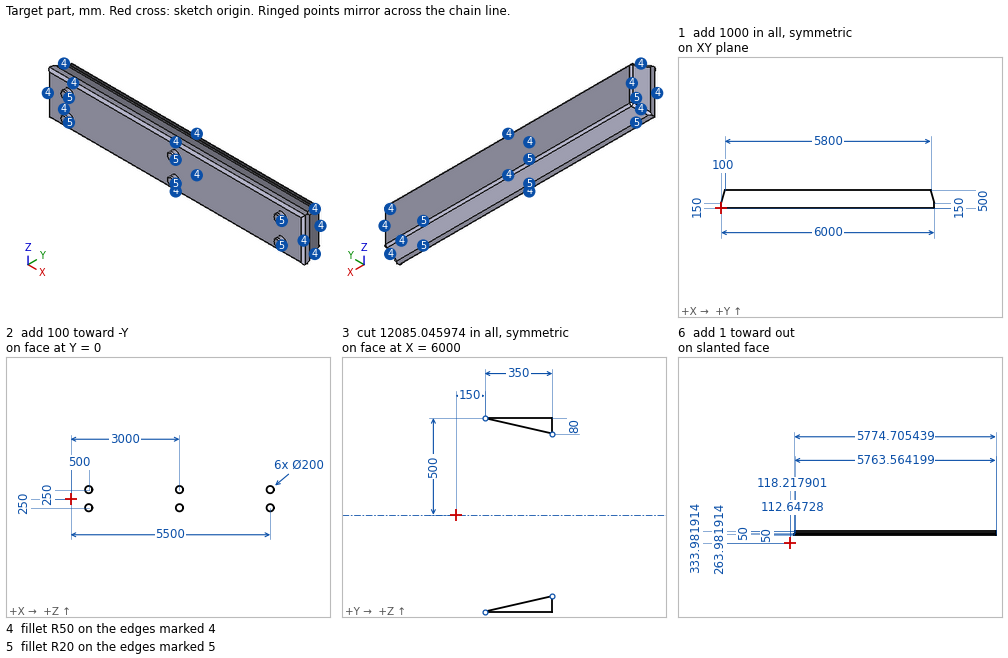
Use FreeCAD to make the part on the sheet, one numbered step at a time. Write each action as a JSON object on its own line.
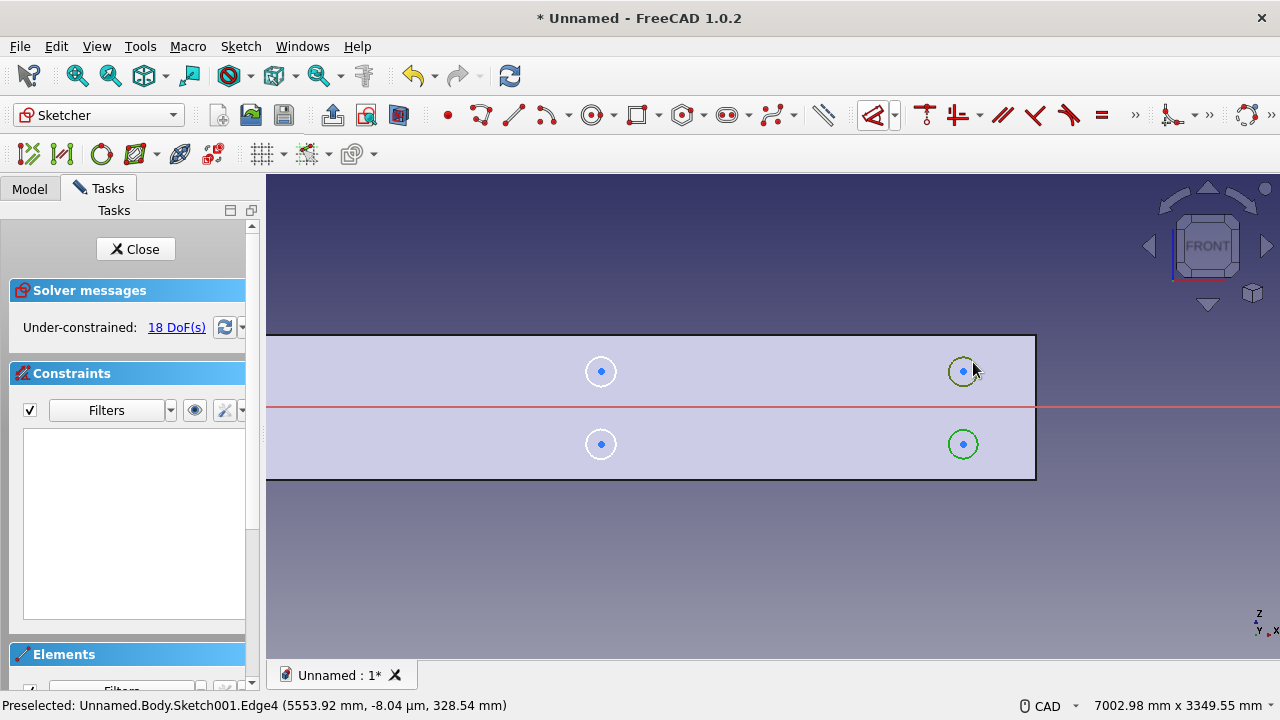
{"action": "left_click", "coordinate": [611, 361]}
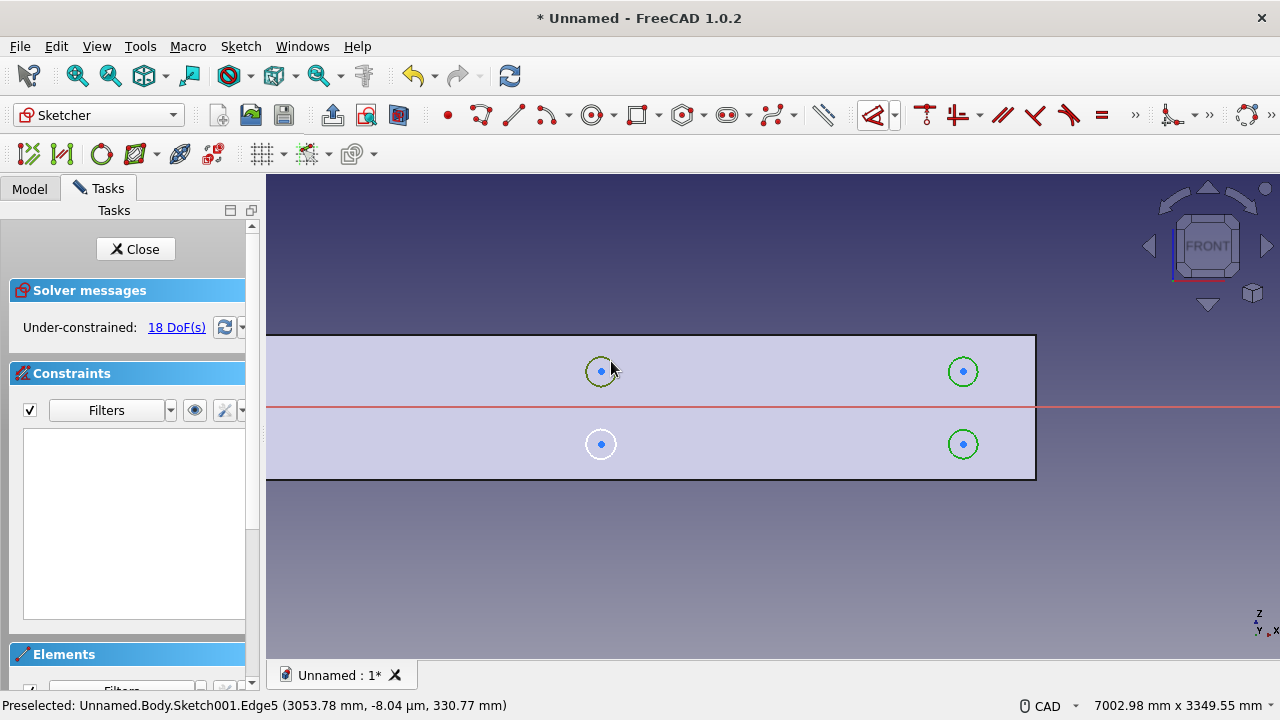
{"action": "left_click", "coordinate": [611, 434]}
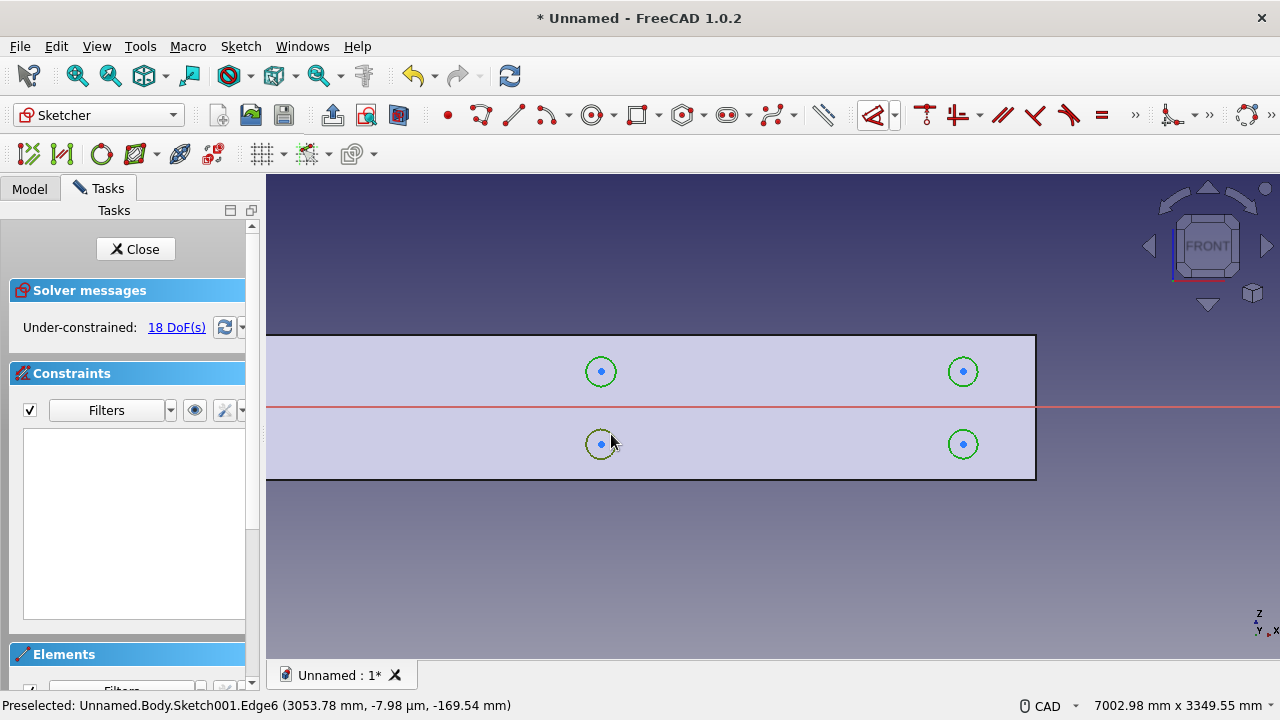
{"action": "left_click", "coordinate": [1102, 116]}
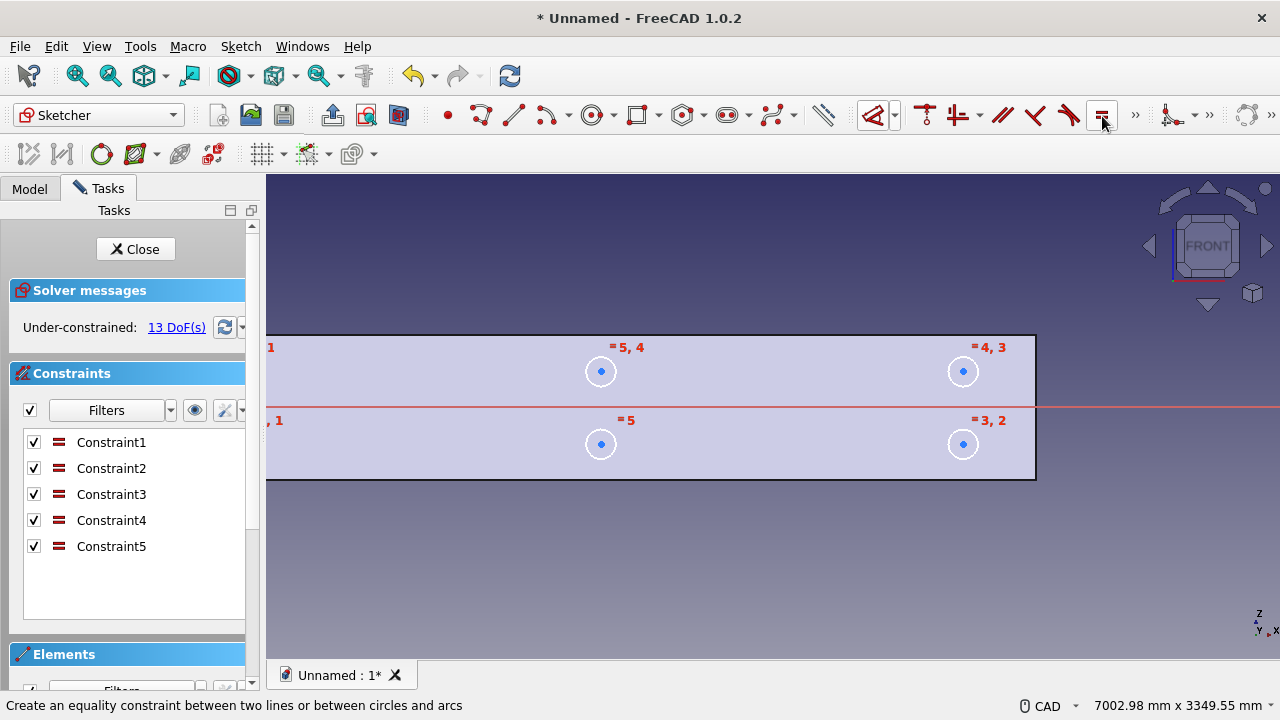
{"action": "scroll", "coordinate": [974, 435], "scroll_direction": "down", "scroll_amount": 2}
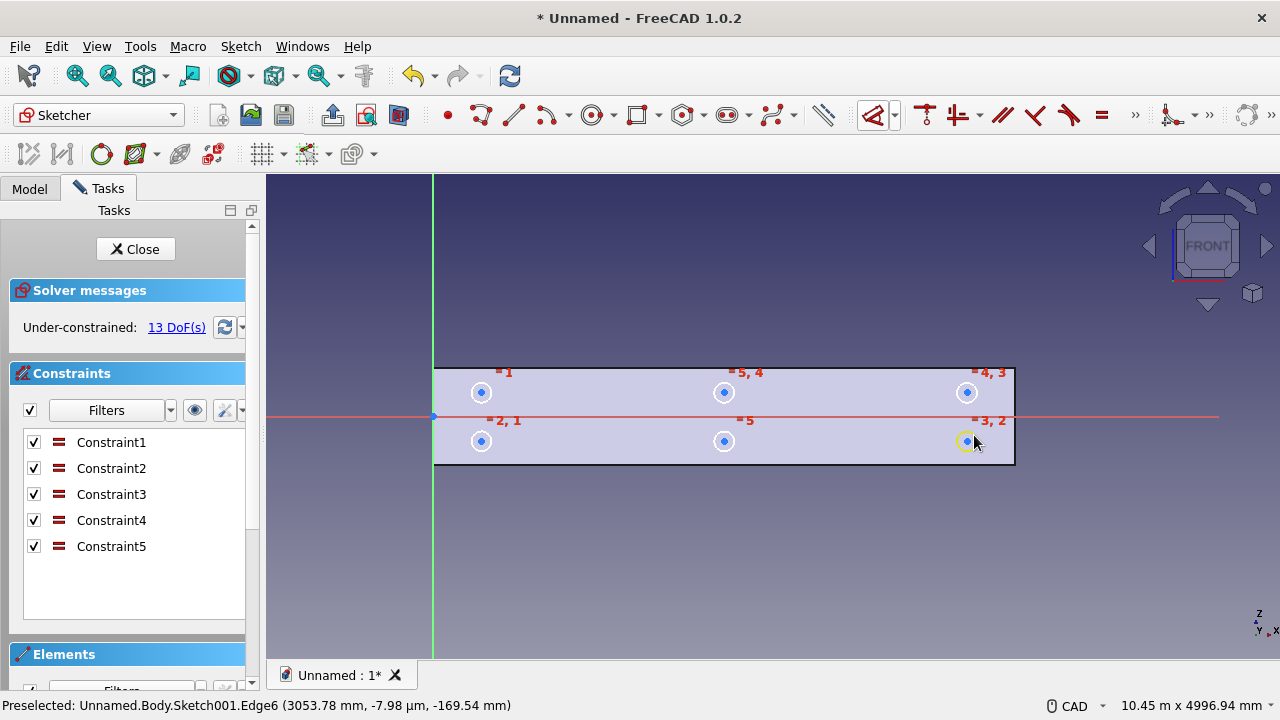
{"action": "left_click", "coordinate": [481, 393]}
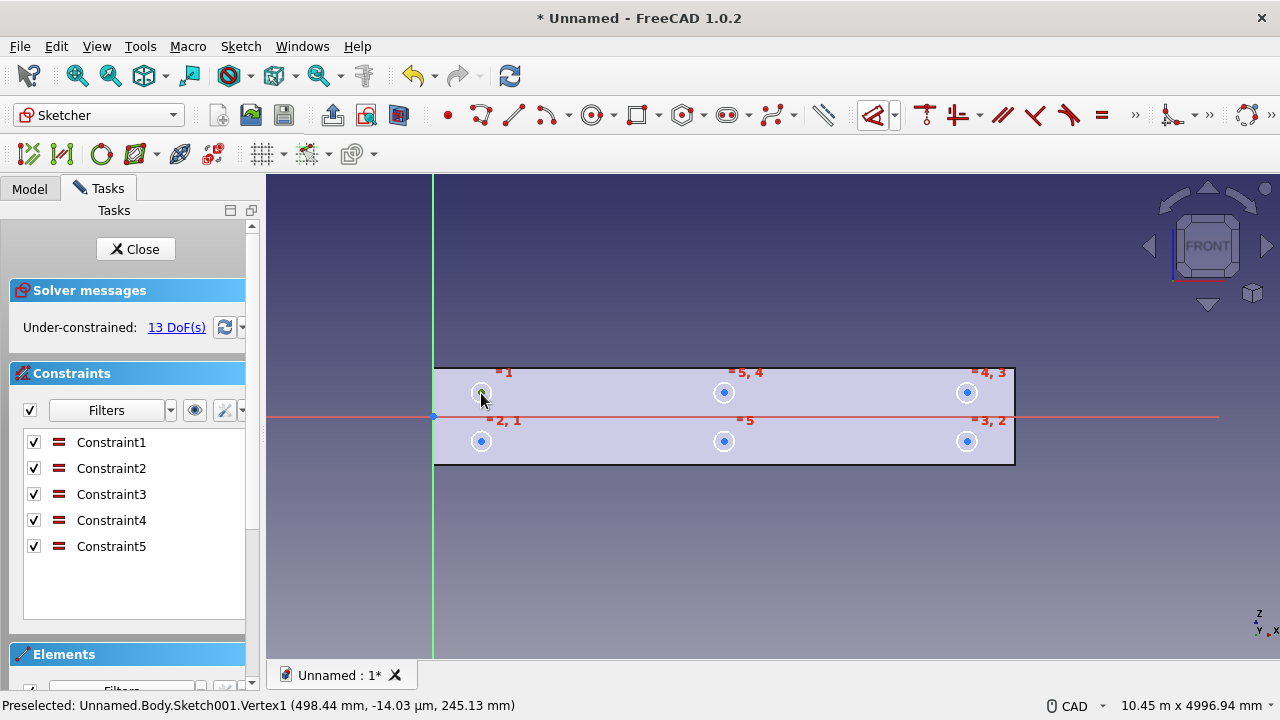
{"action": "left_click", "coordinate": [481, 441]}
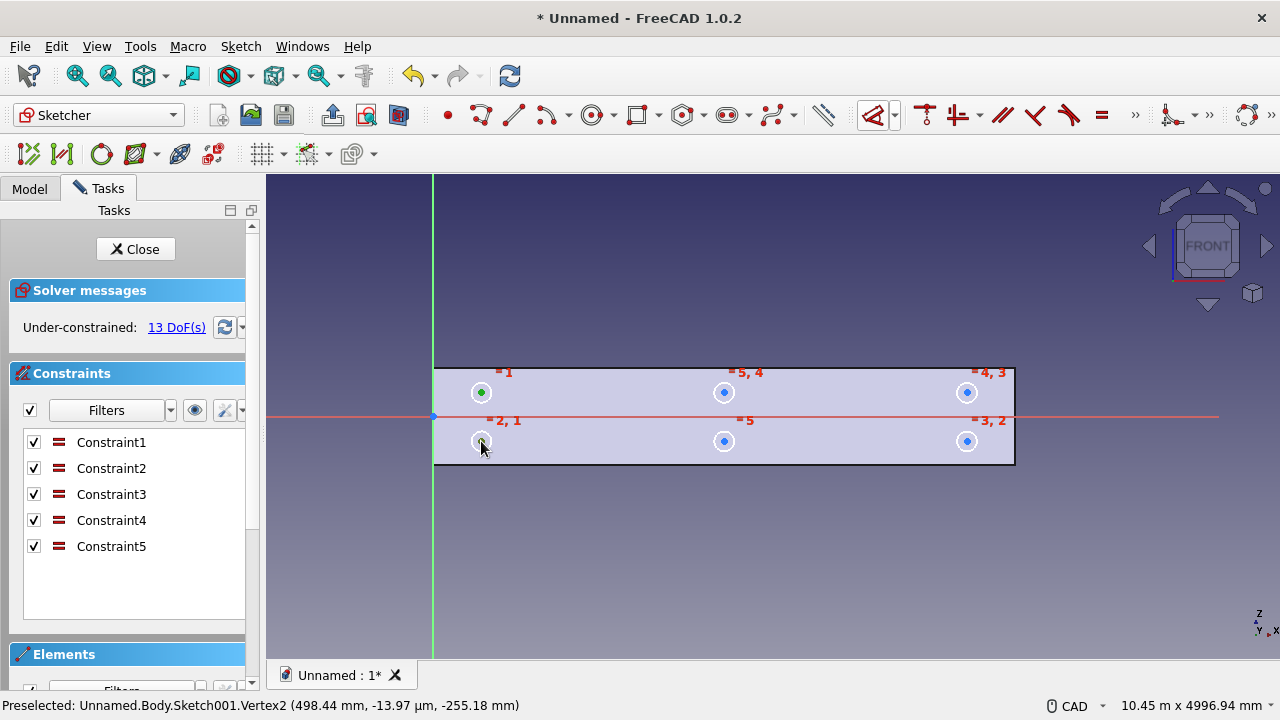
{"action": "left_click", "coordinate": [980, 116]}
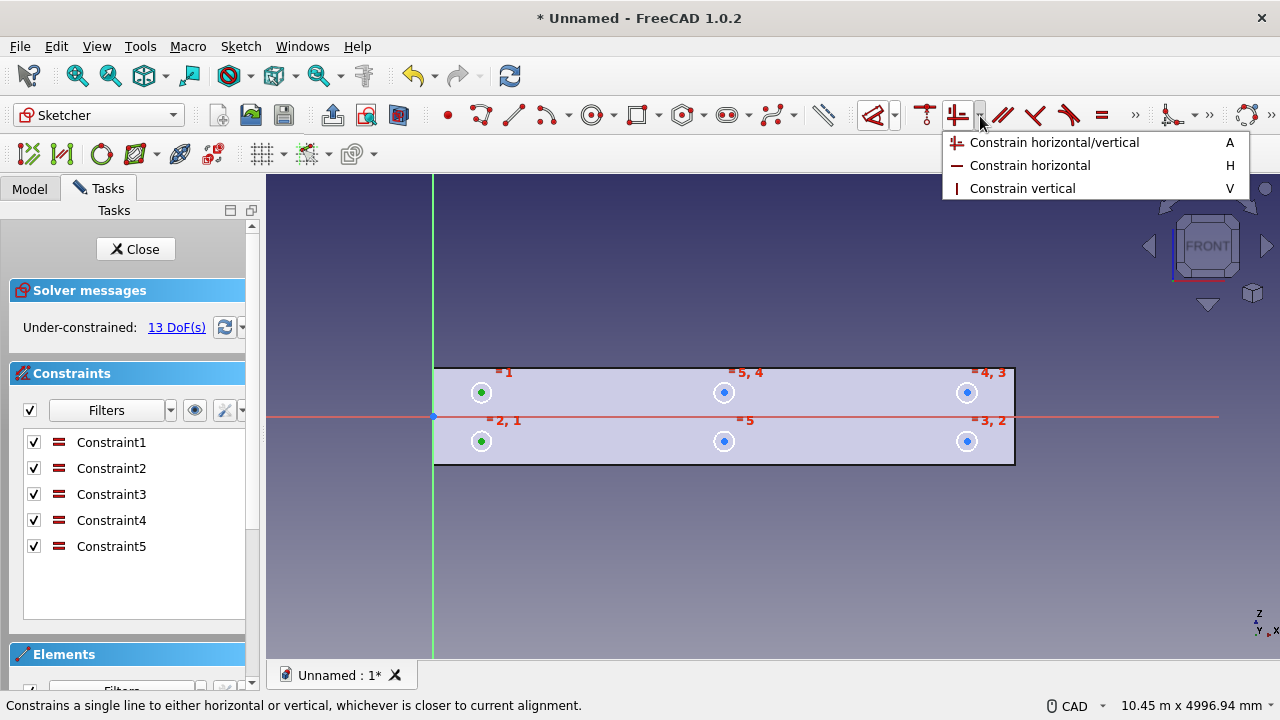
{"action": "left_click", "coordinate": [1096, 188]}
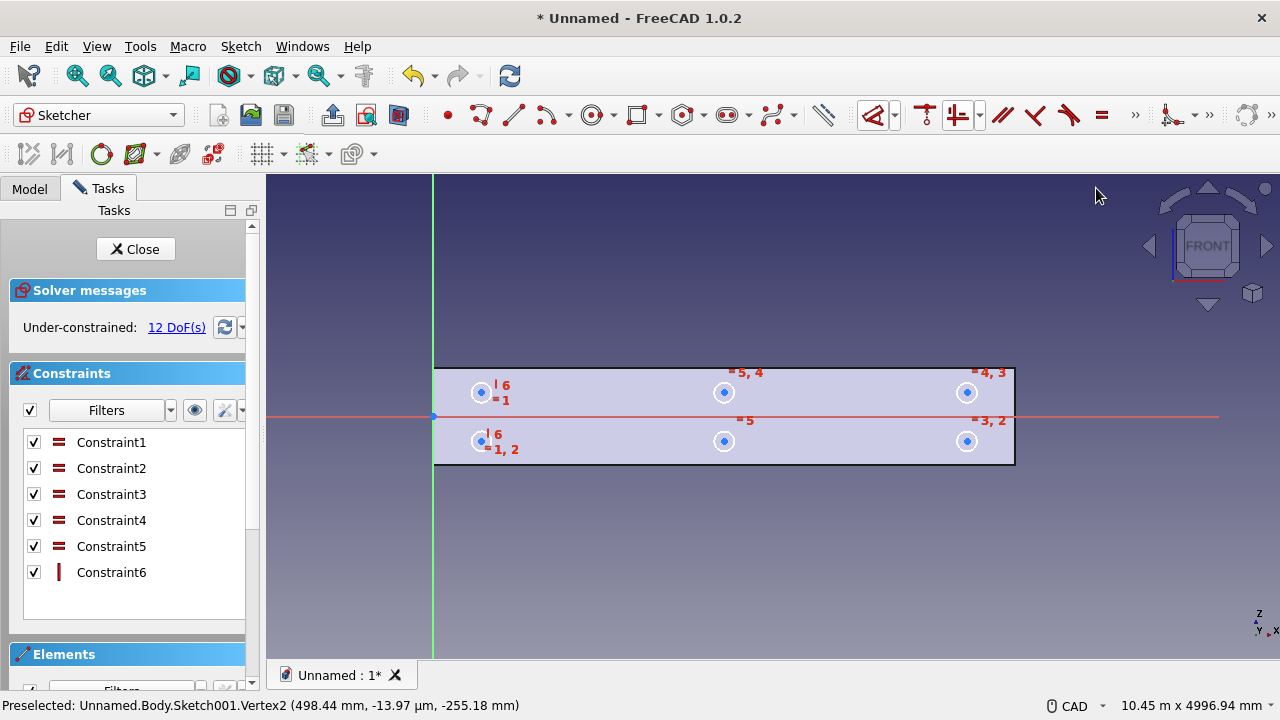
{"action": "left_click", "coordinate": [481, 441]}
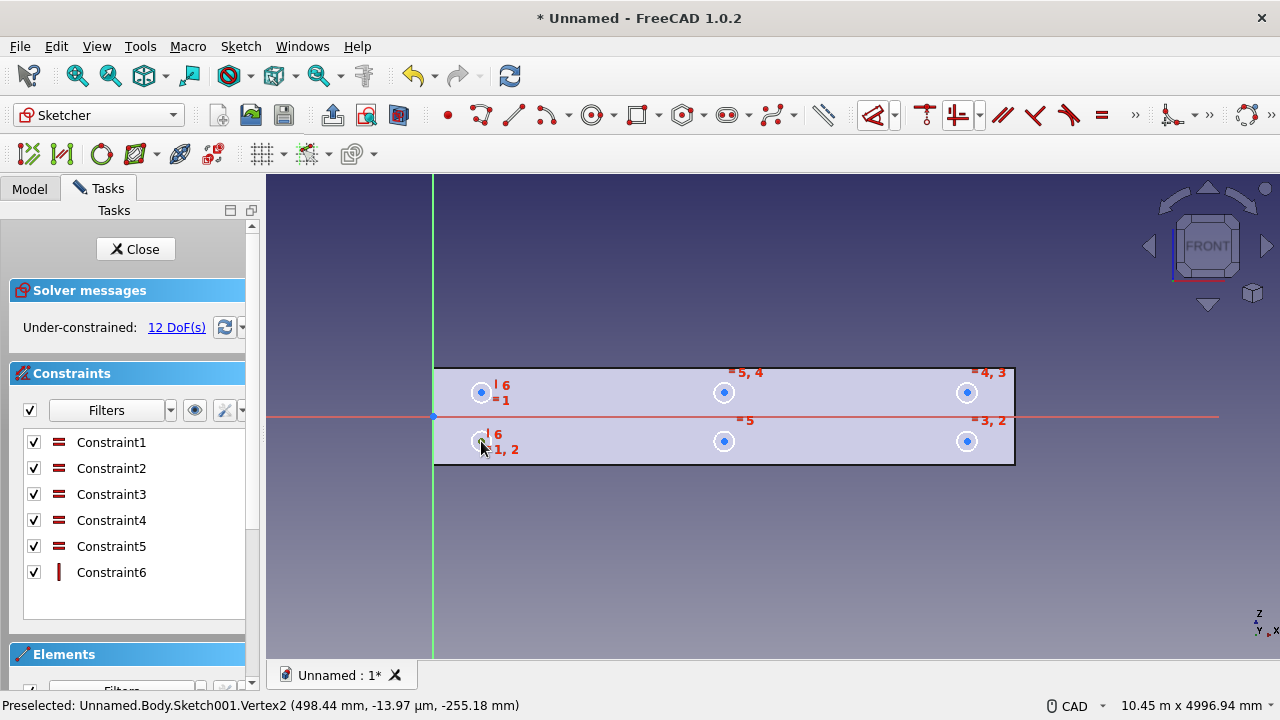
{"action": "left_click", "coordinate": [967, 441]}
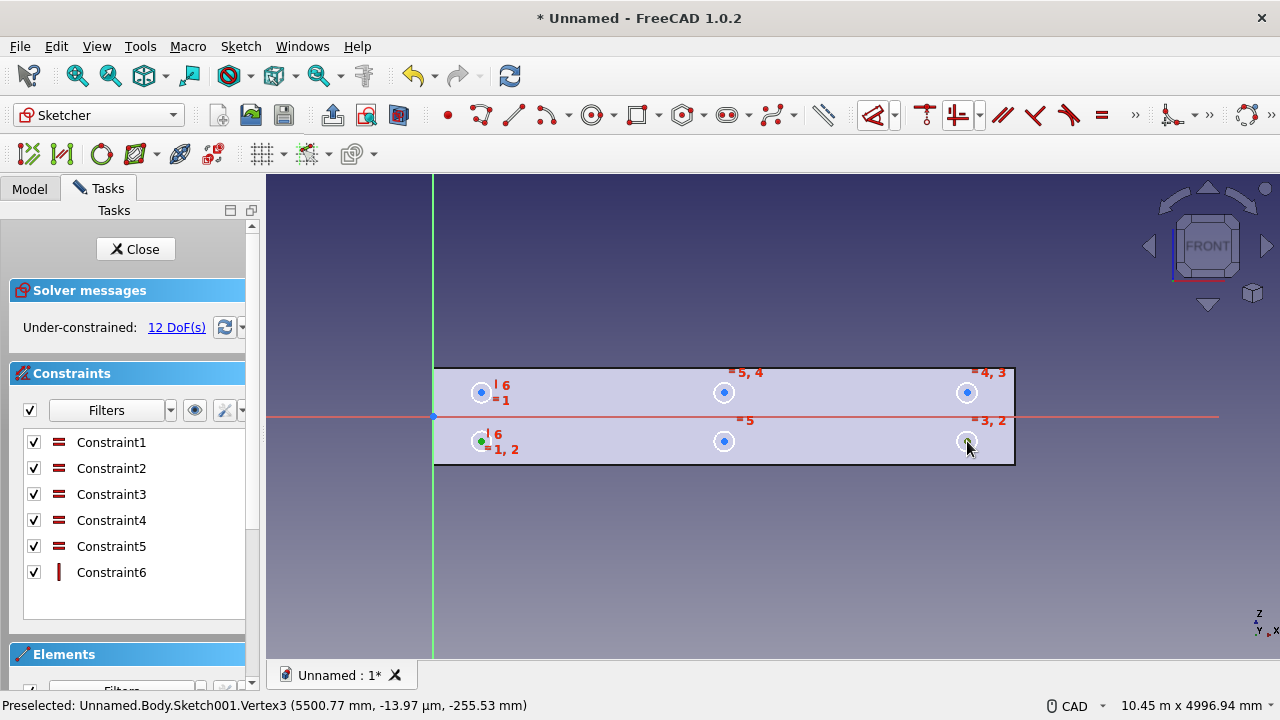
{"action": "left_click", "coordinate": [980, 116]}